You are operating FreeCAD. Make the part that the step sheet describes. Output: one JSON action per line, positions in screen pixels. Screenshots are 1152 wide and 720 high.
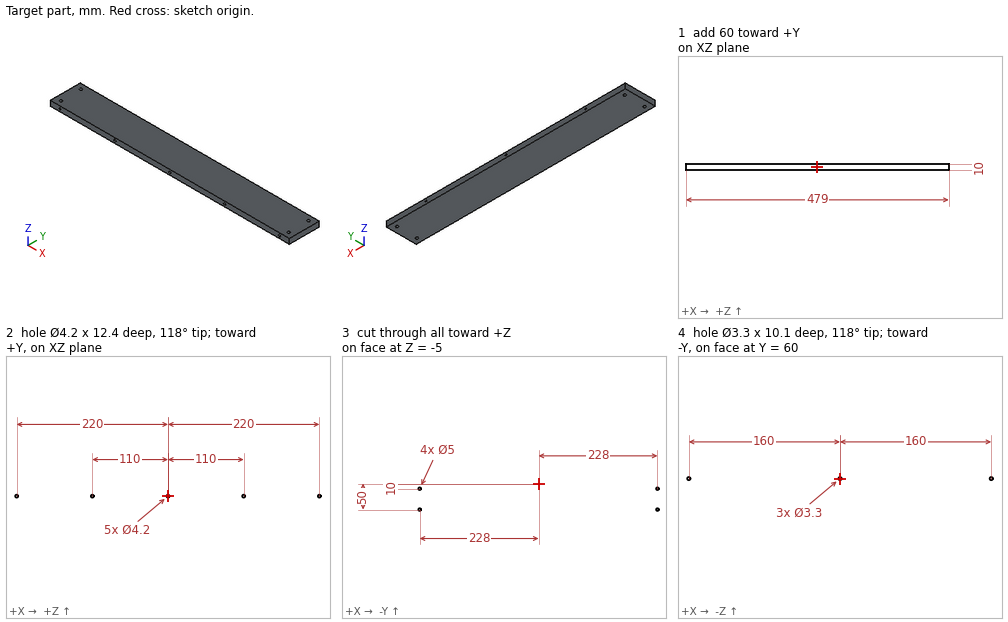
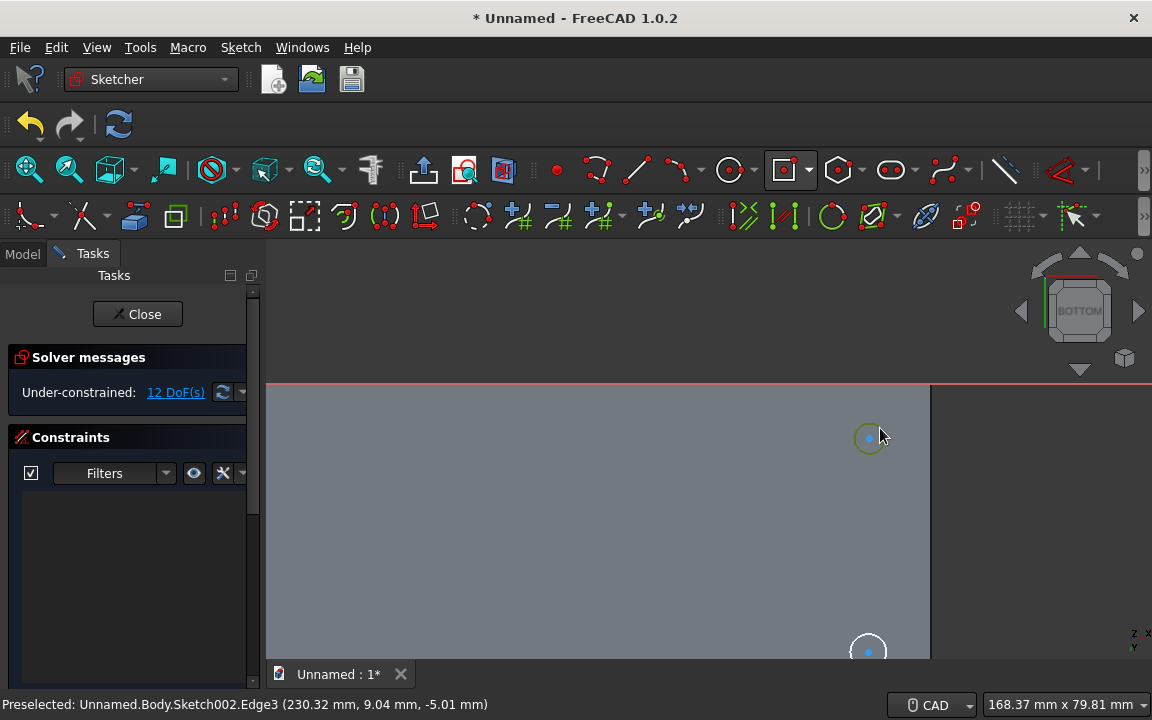
{"action": "scroll", "coordinate": [886, 431], "scroll_direction": "down", "scroll_amount": 8}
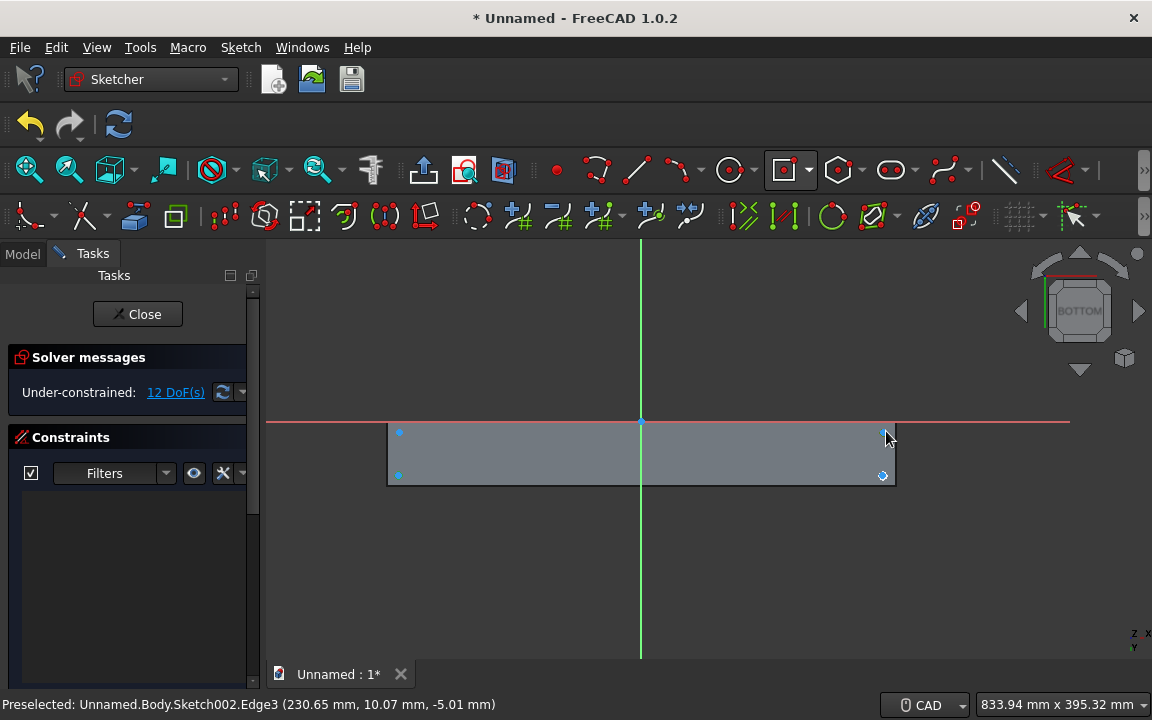
{"action": "scroll", "coordinate": [886, 473], "scroll_direction": "up", "scroll_amount": 7}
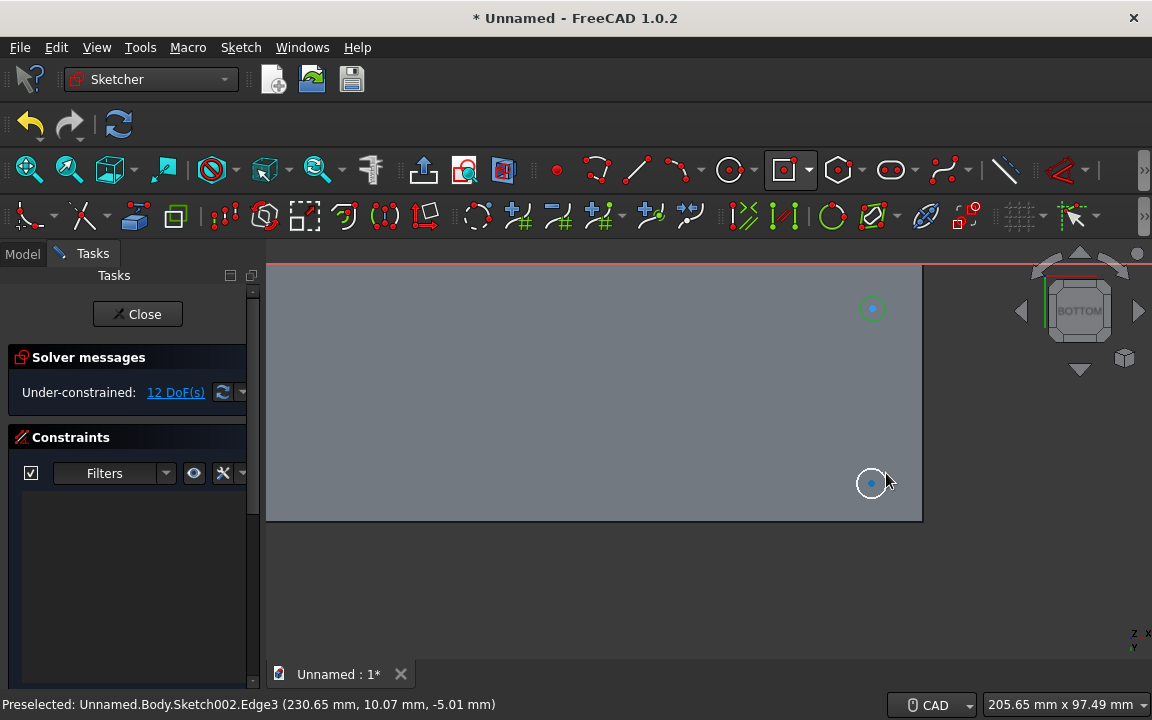
{"action": "left_click", "coordinate": [882, 473]}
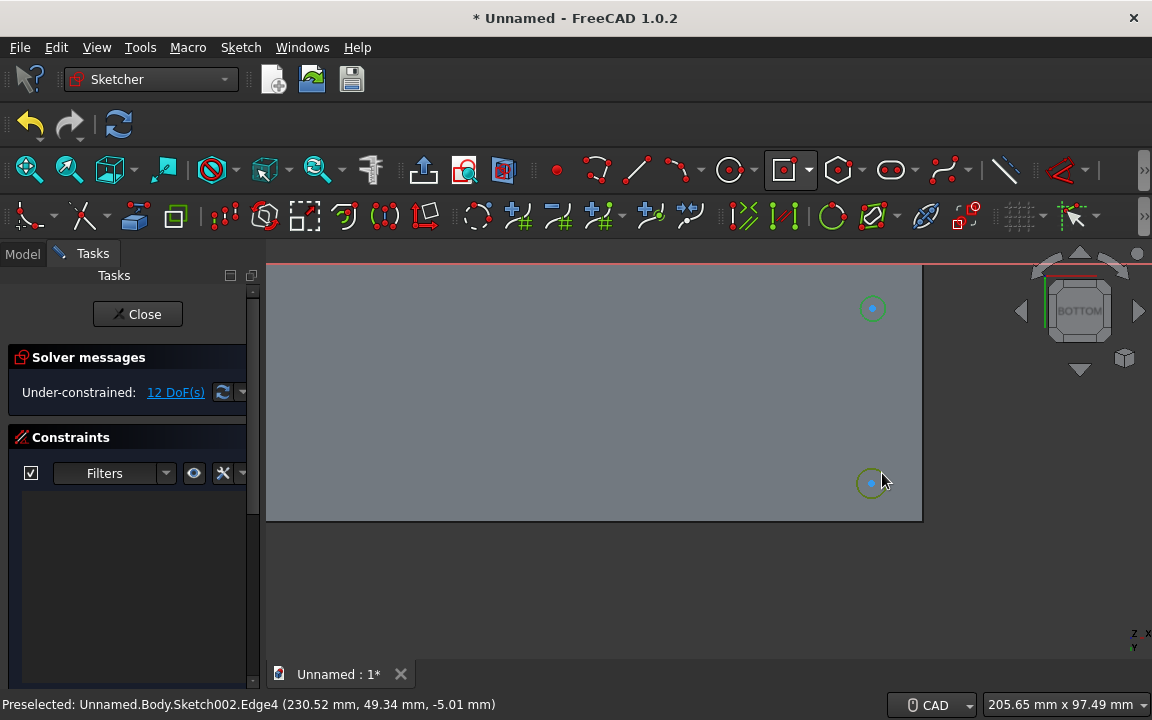
{"action": "key", "text": "e"}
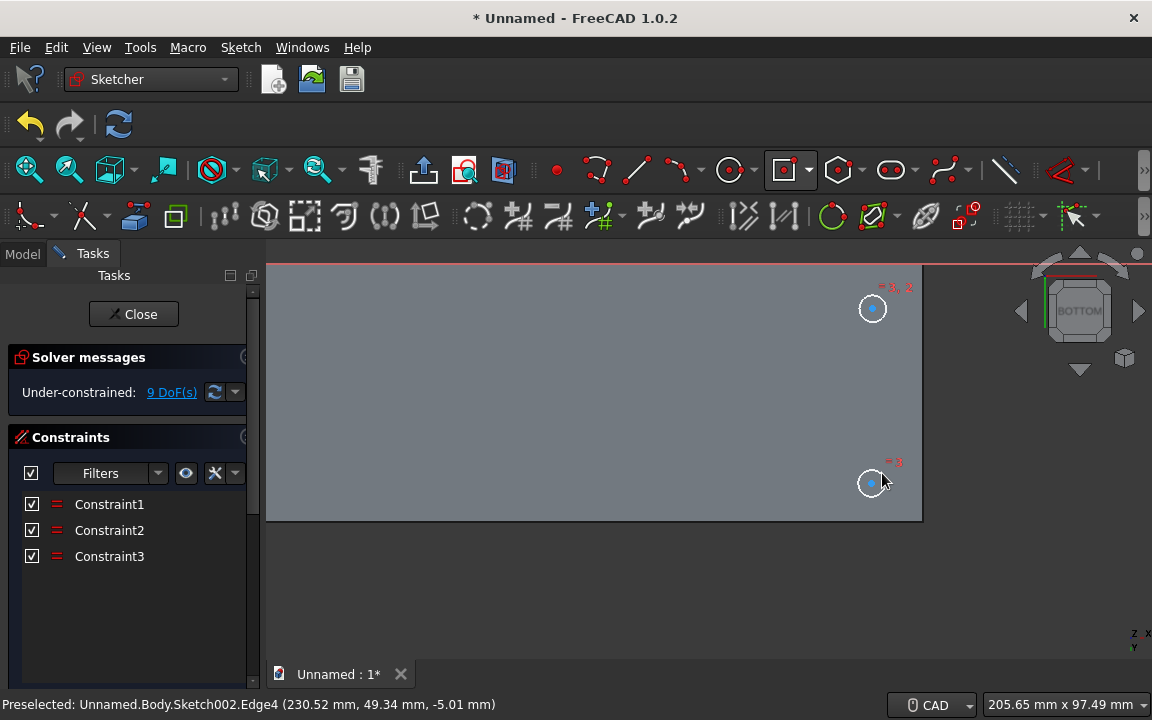
{"action": "scroll", "coordinate": [886, 473], "scroll_direction": "down", "scroll_amount": 7}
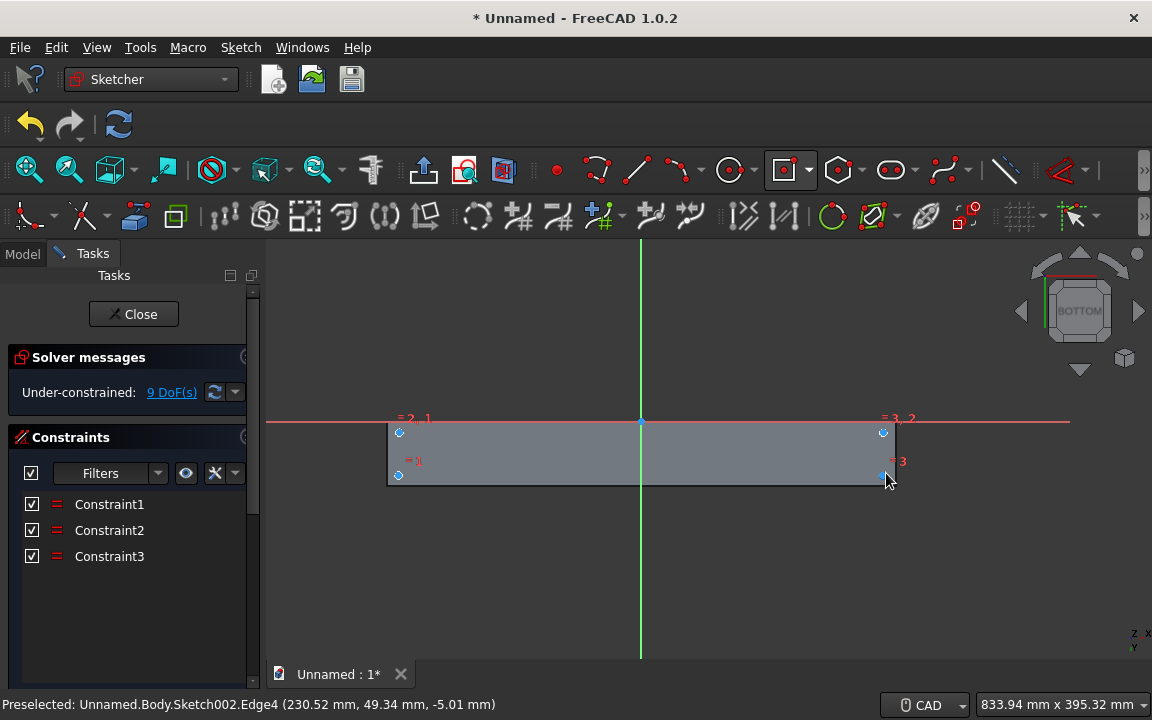
{"action": "left_click", "coordinate": [399, 476]}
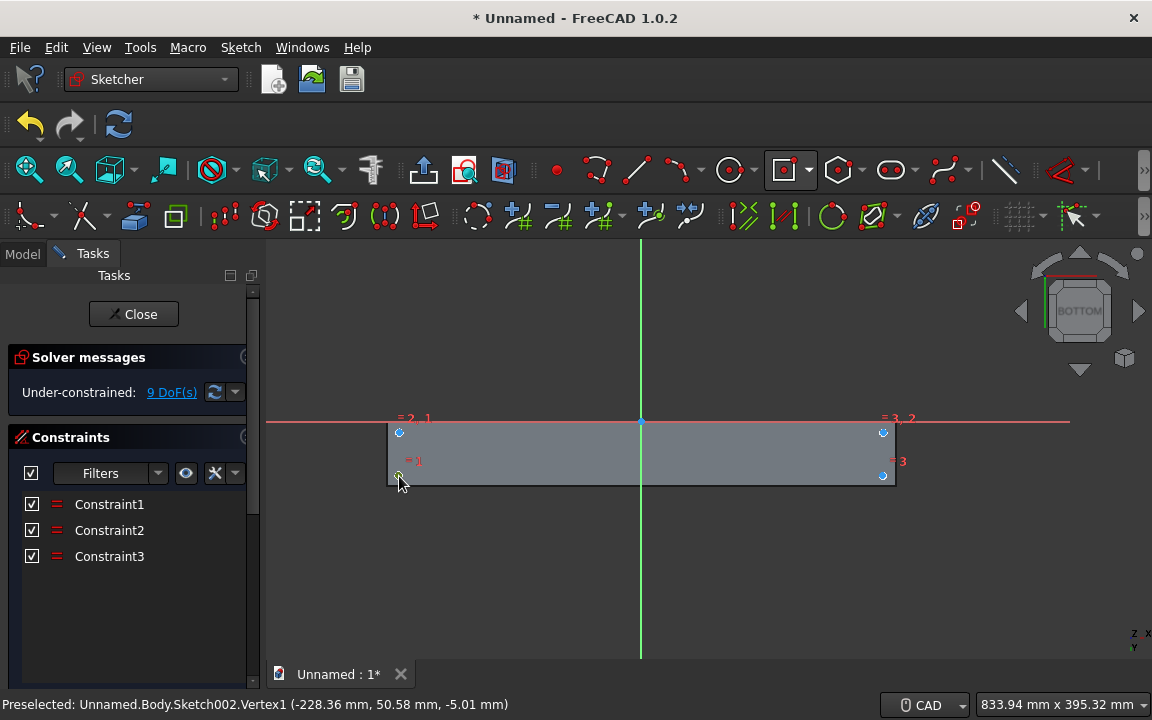
{"action": "left_click", "coordinate": [399, 433]}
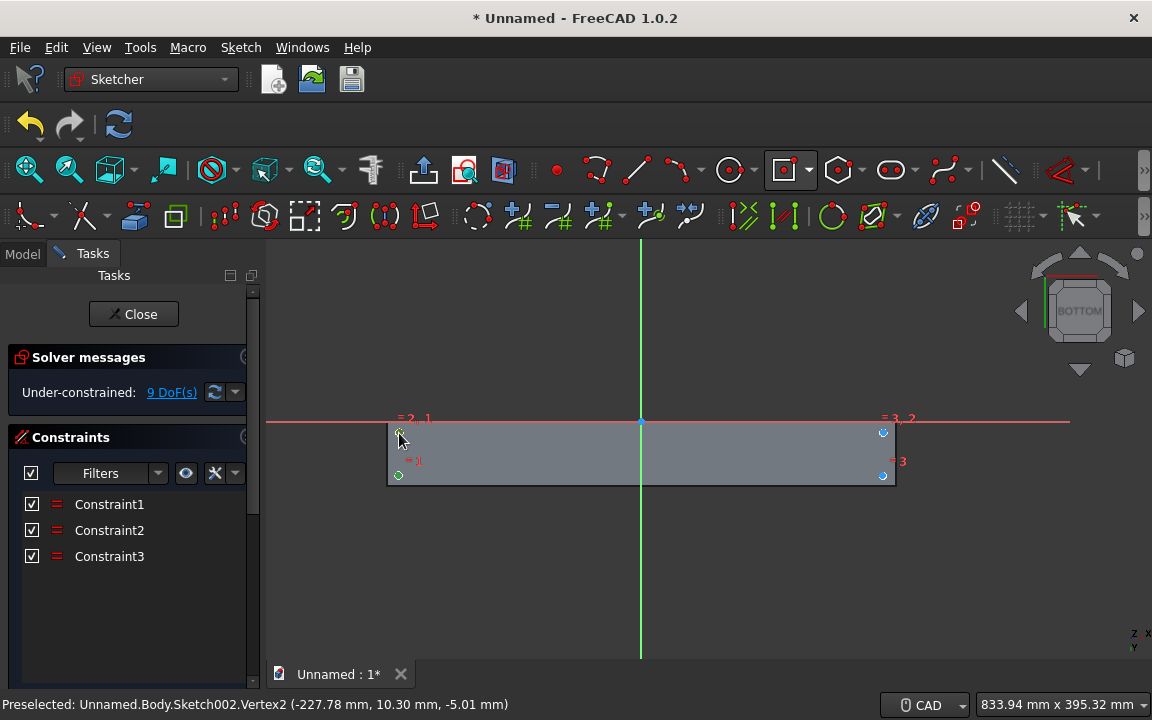
{"action": "key", "text": "v"}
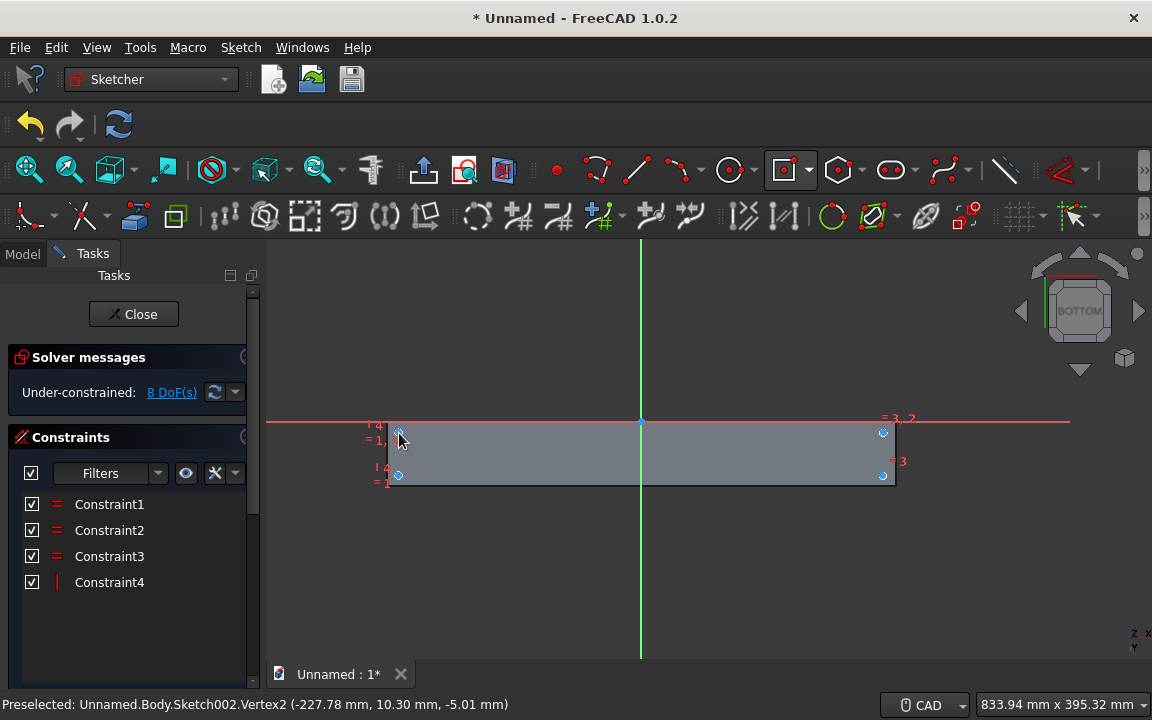
{"action": "left_click", "coordinate": [401, 435]}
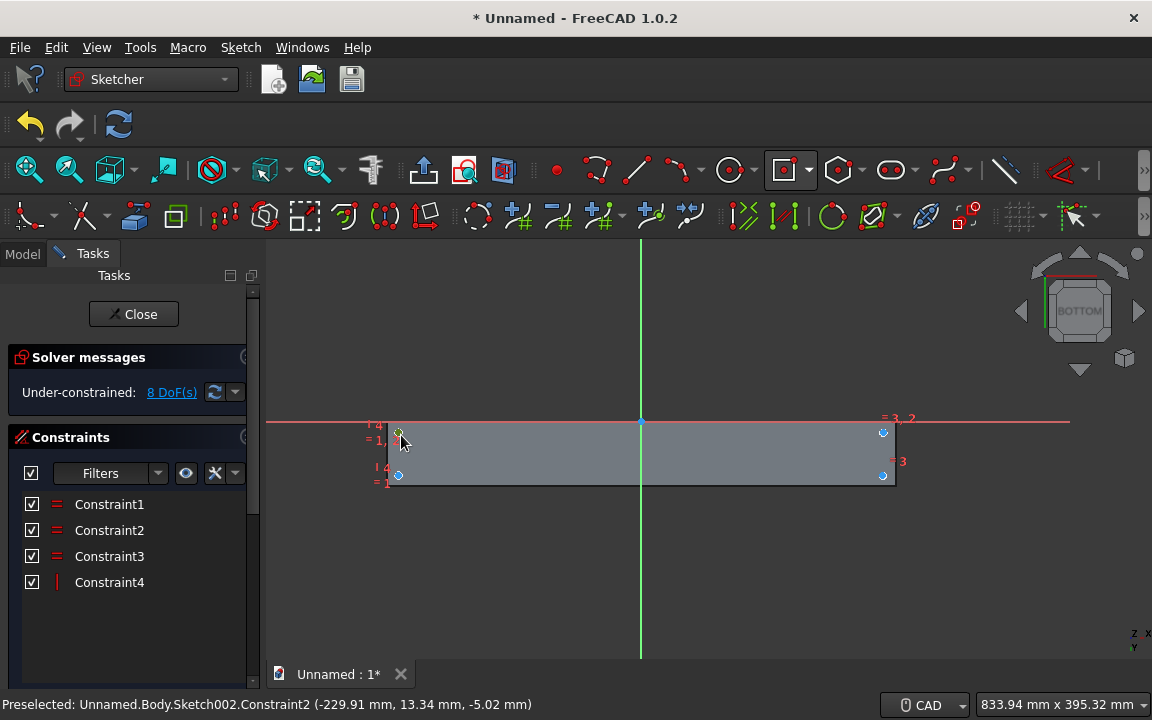
{"action": "left_click", "coordinate": [883, 433]}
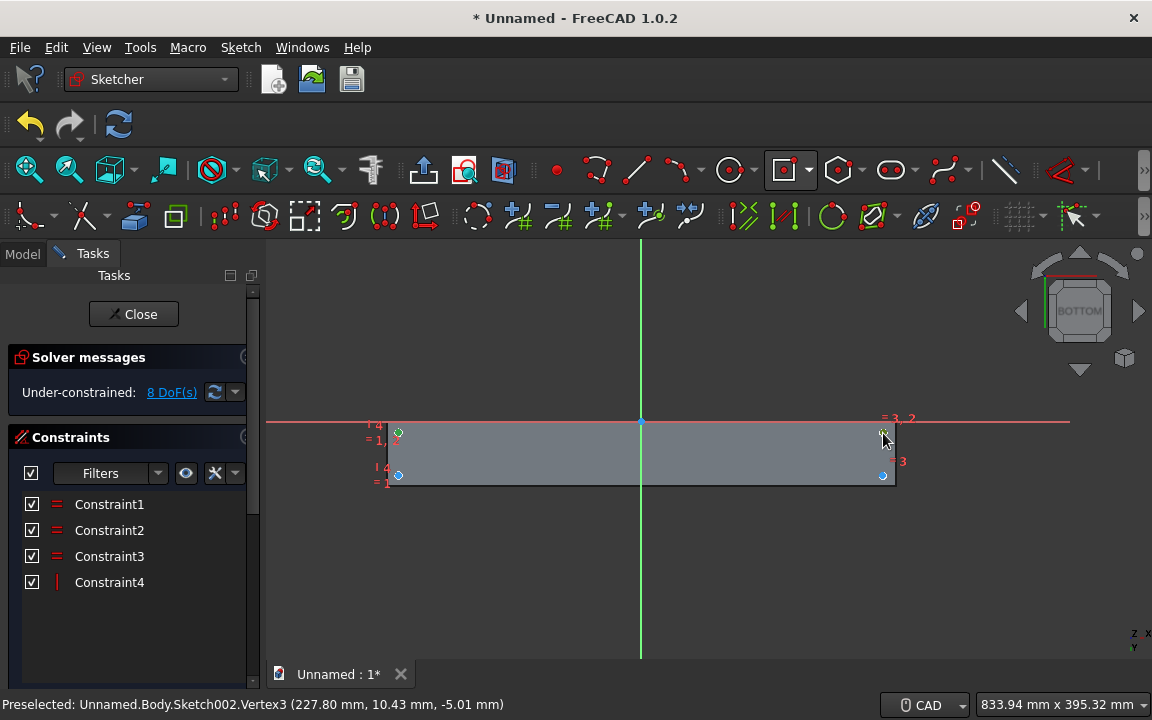
{"action": "key", "text": "h"}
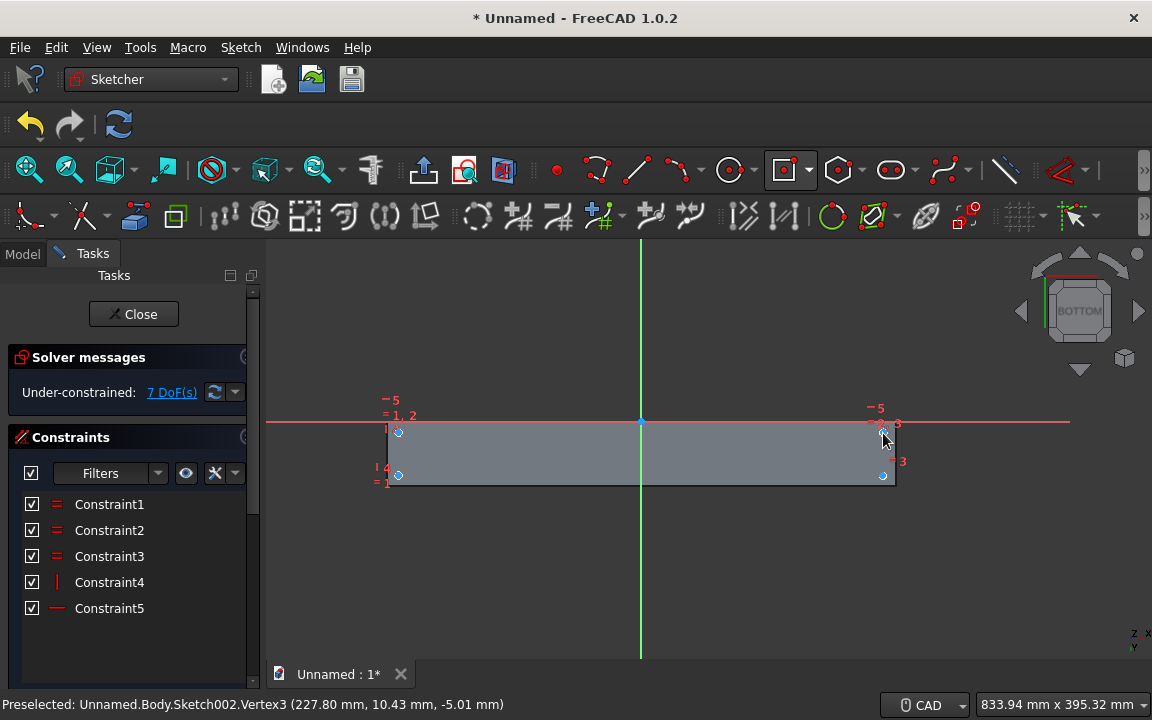
{"action": "left_click", "coordinate": [883, 433]}